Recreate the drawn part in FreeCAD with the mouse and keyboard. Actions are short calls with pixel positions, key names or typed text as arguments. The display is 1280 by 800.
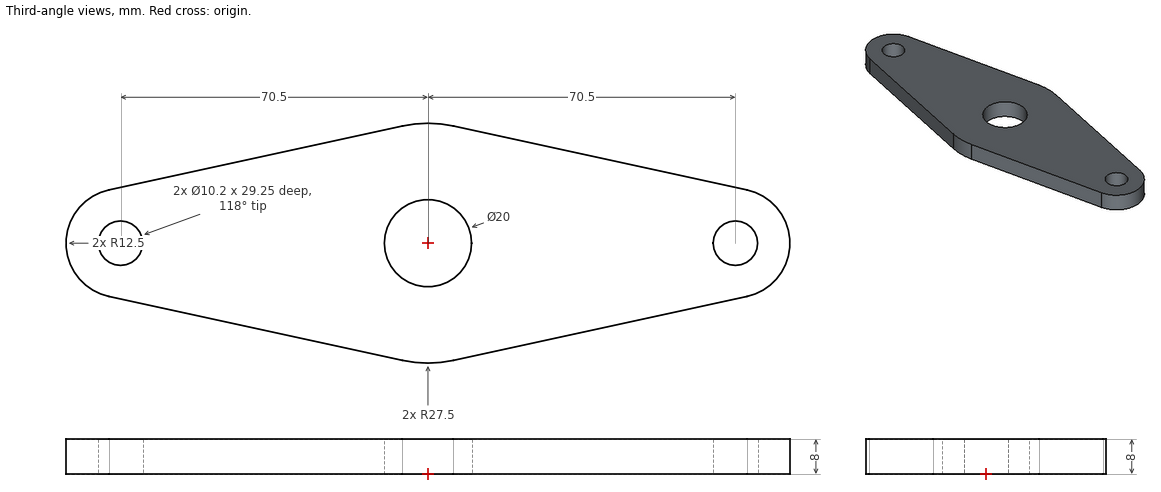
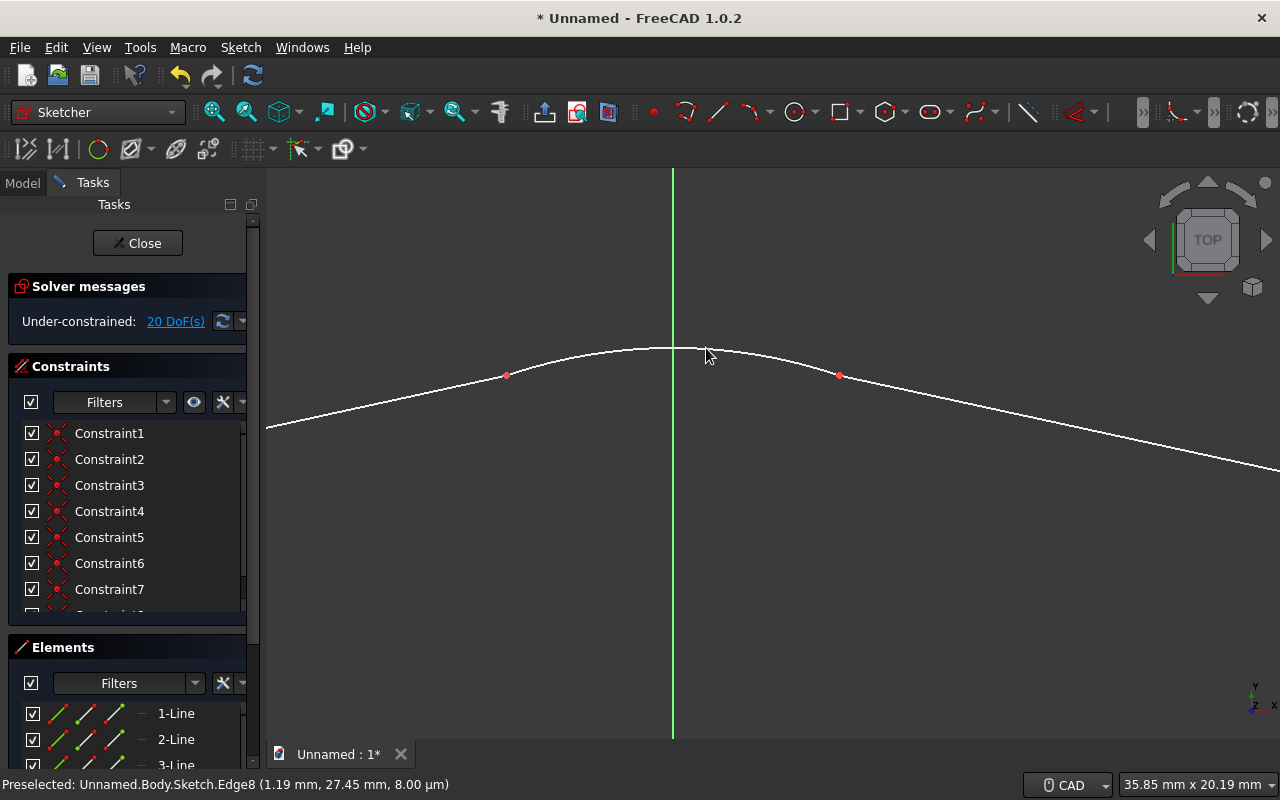
scroll(709, 348, down, 10)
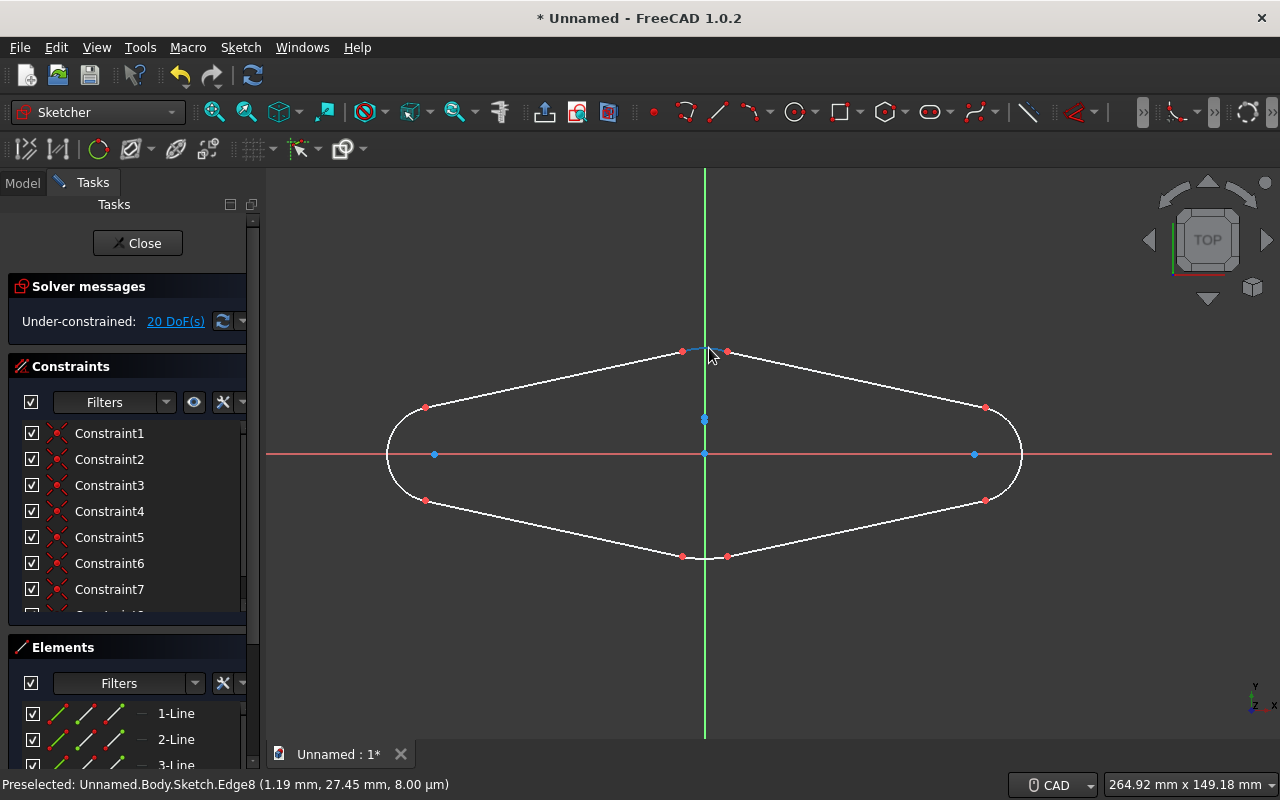
click(605, 369)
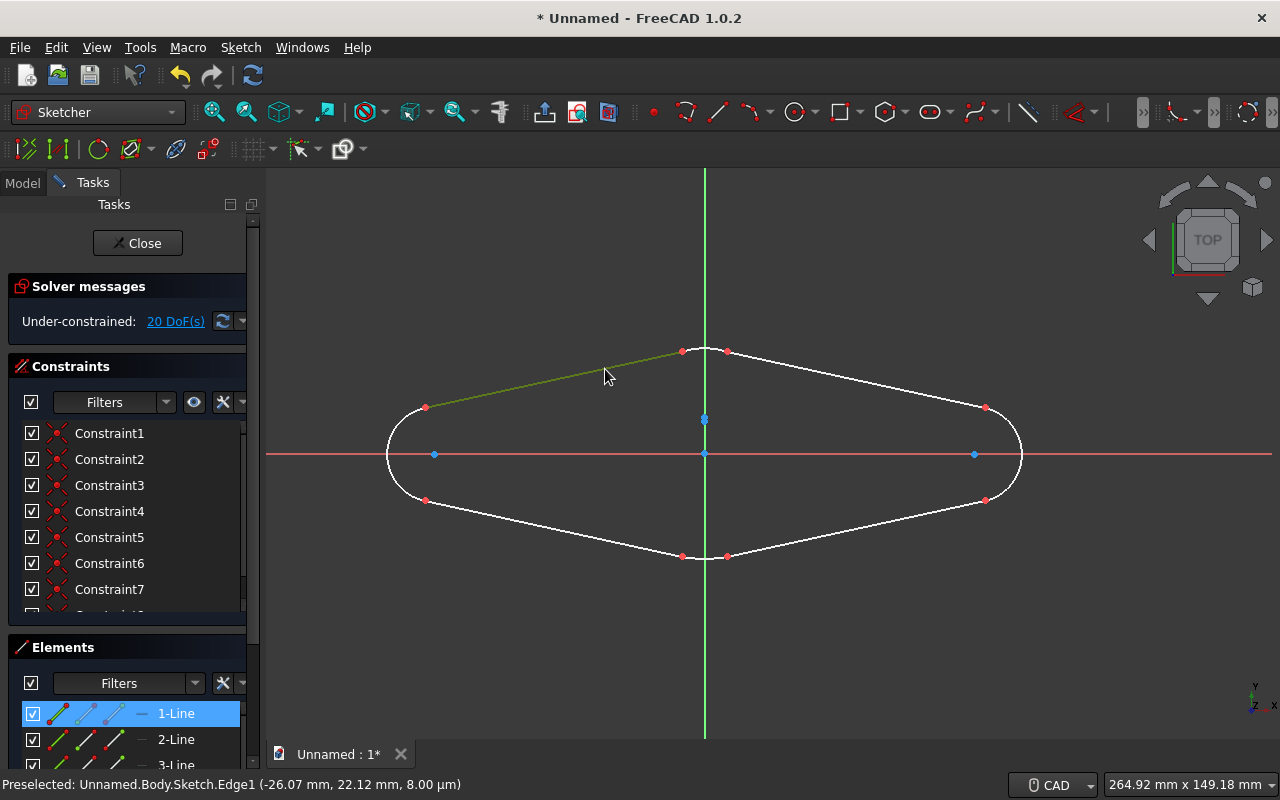
click(394, 430)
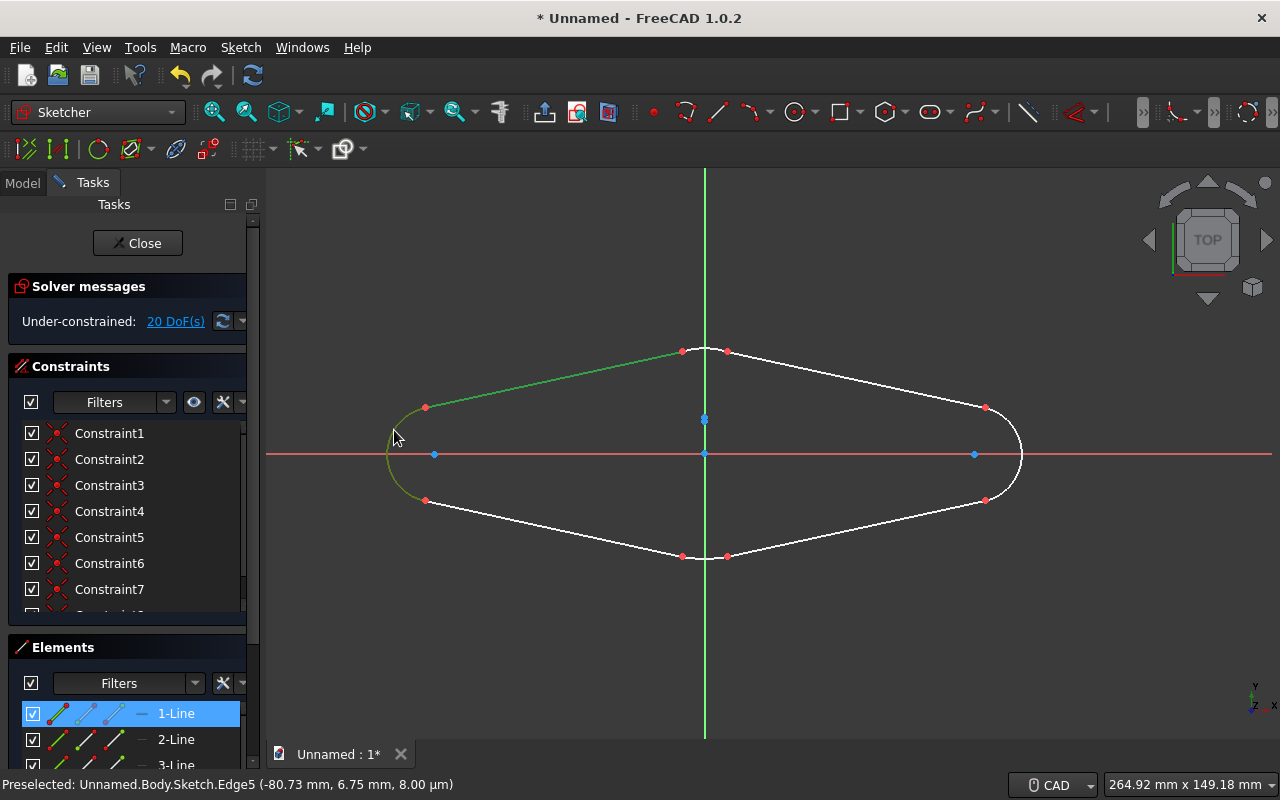
key(t)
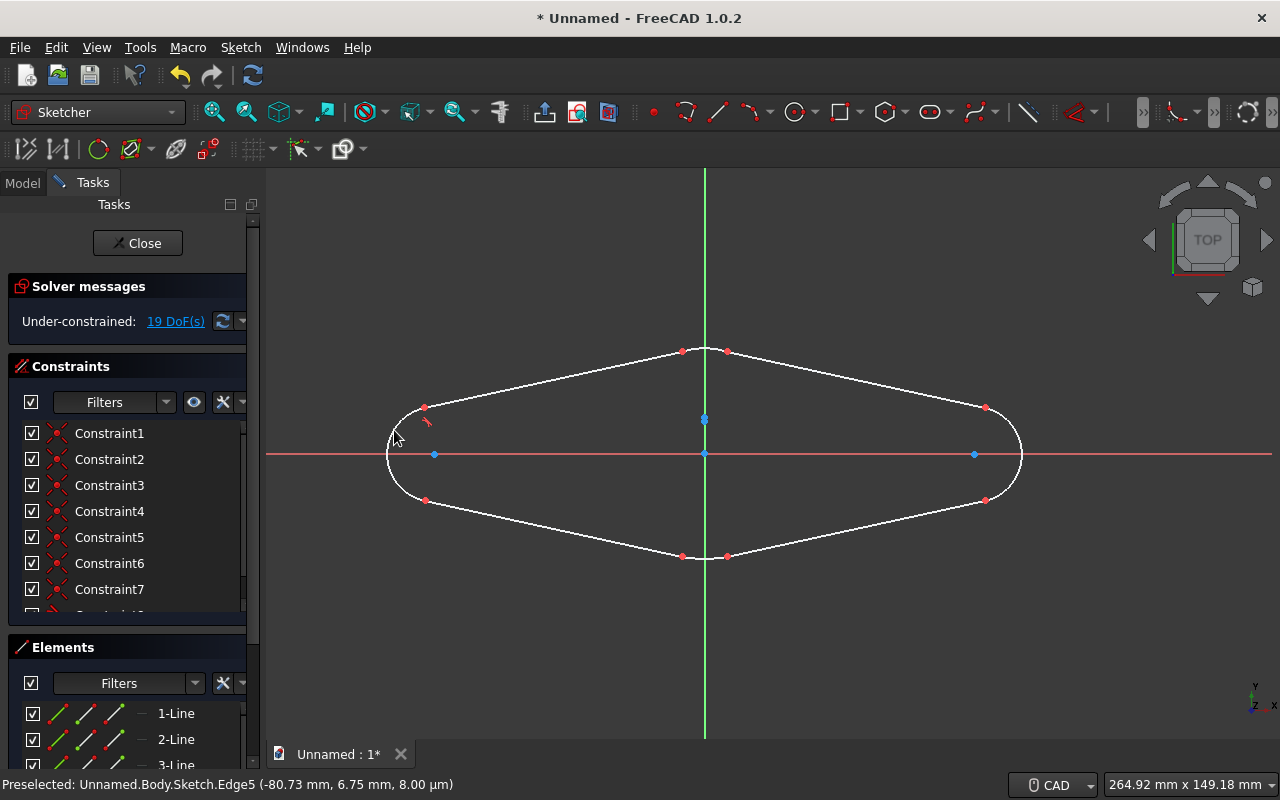
click(605, 369)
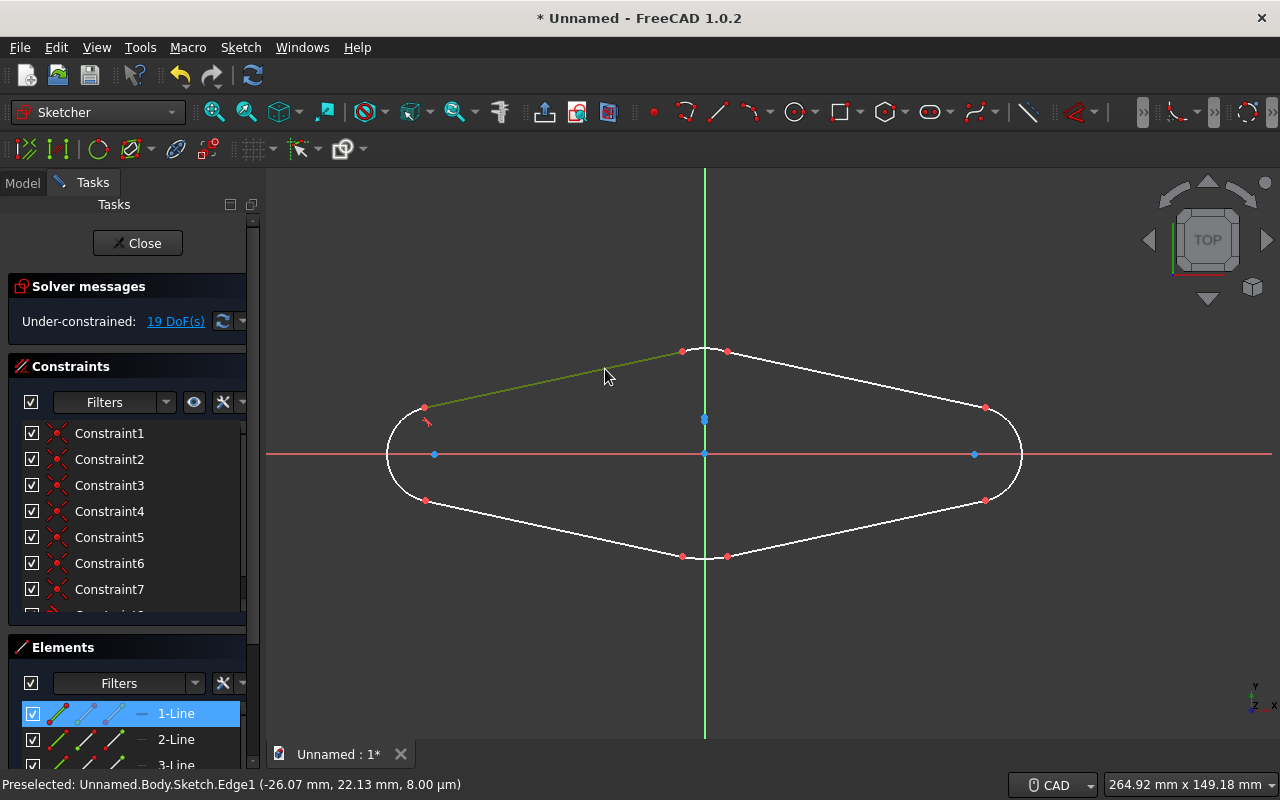
scroll(714, 349, up, 3)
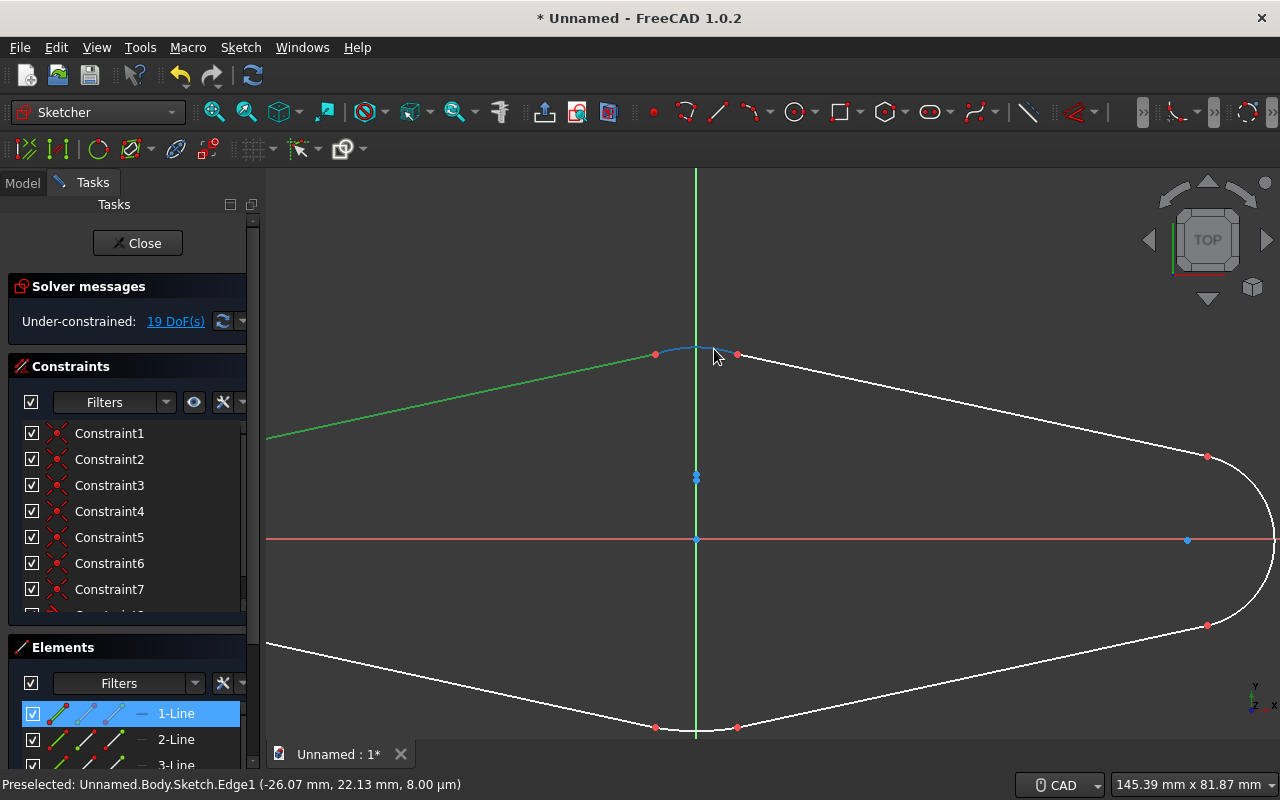
click(713, 348)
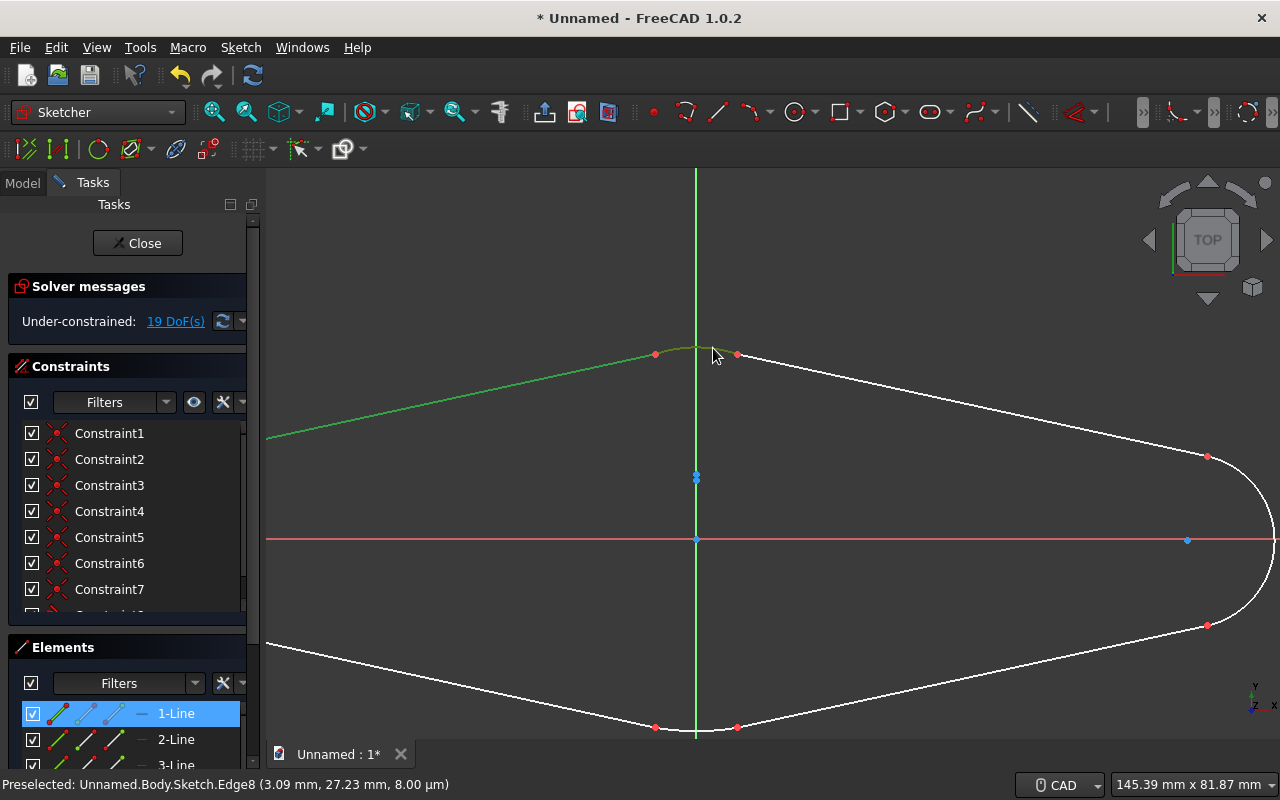
key(t)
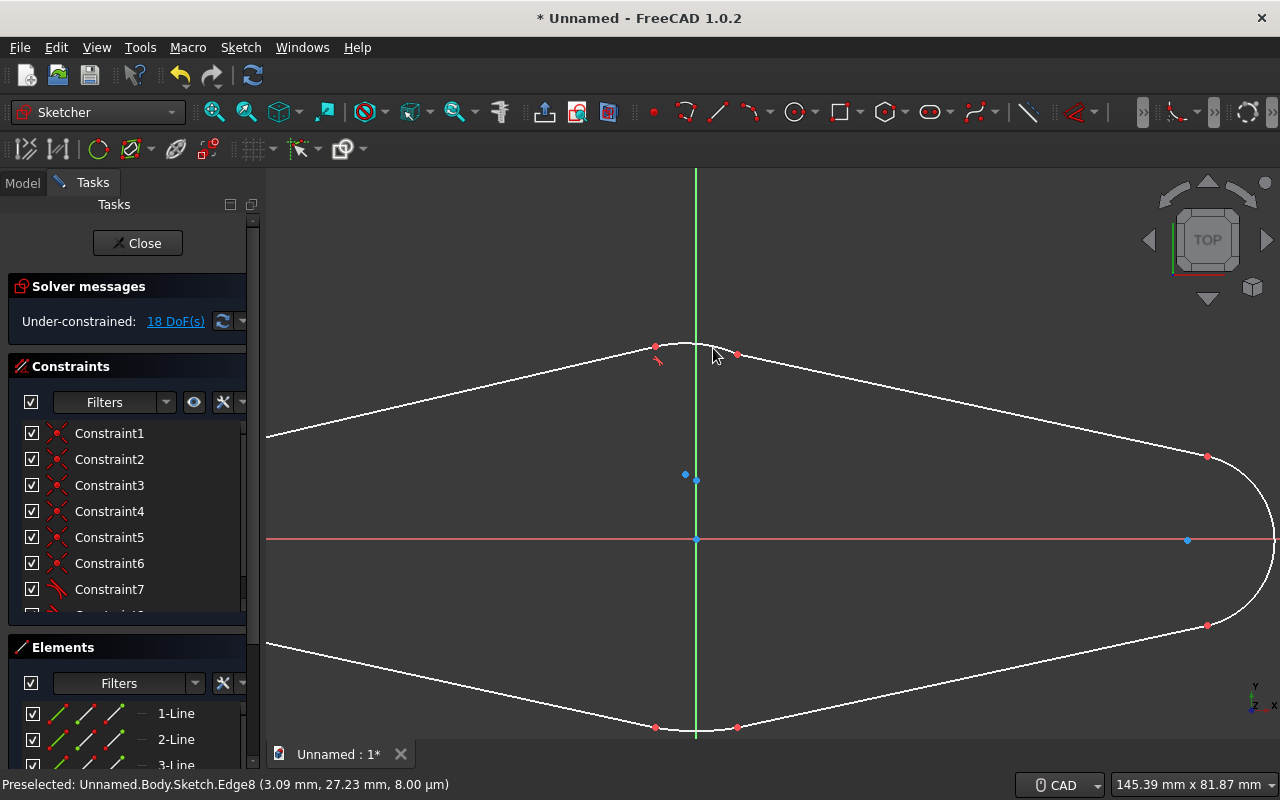
click(328, 656)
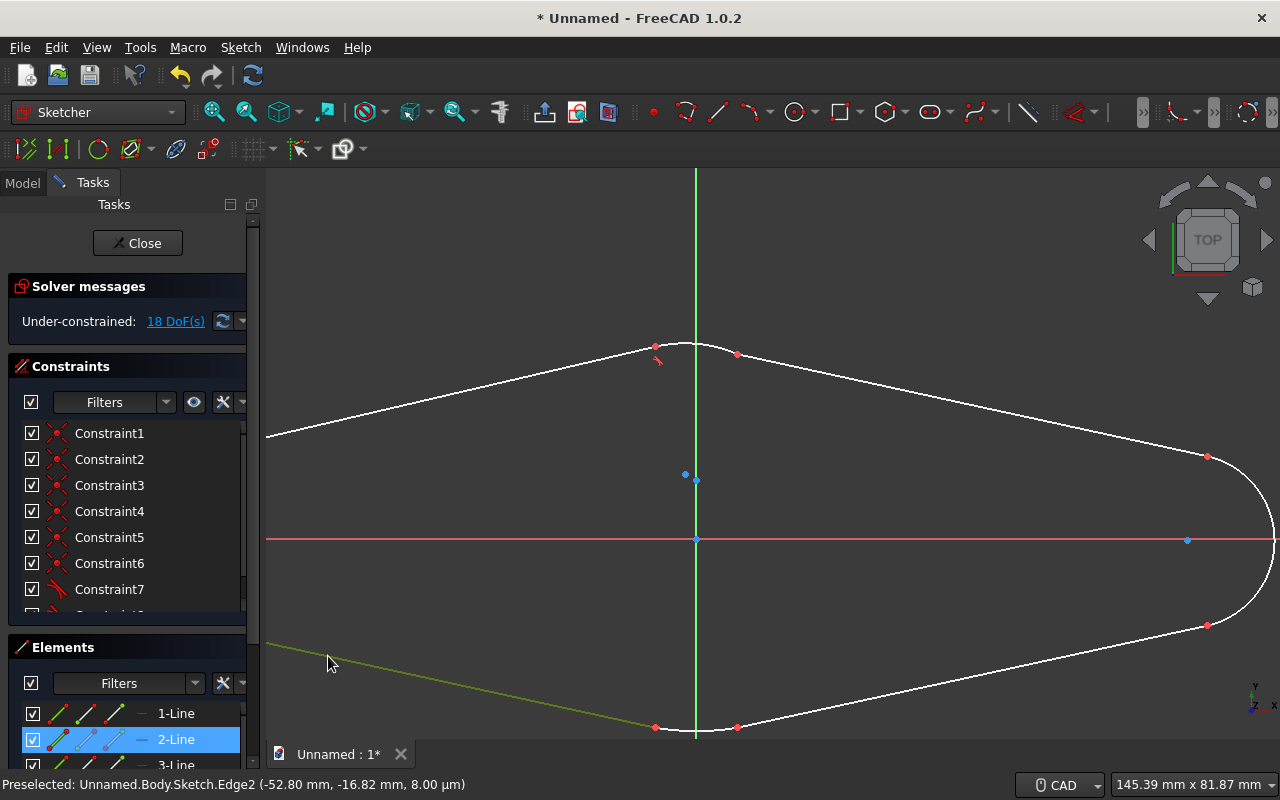
scroll(714, 349, down, 3)